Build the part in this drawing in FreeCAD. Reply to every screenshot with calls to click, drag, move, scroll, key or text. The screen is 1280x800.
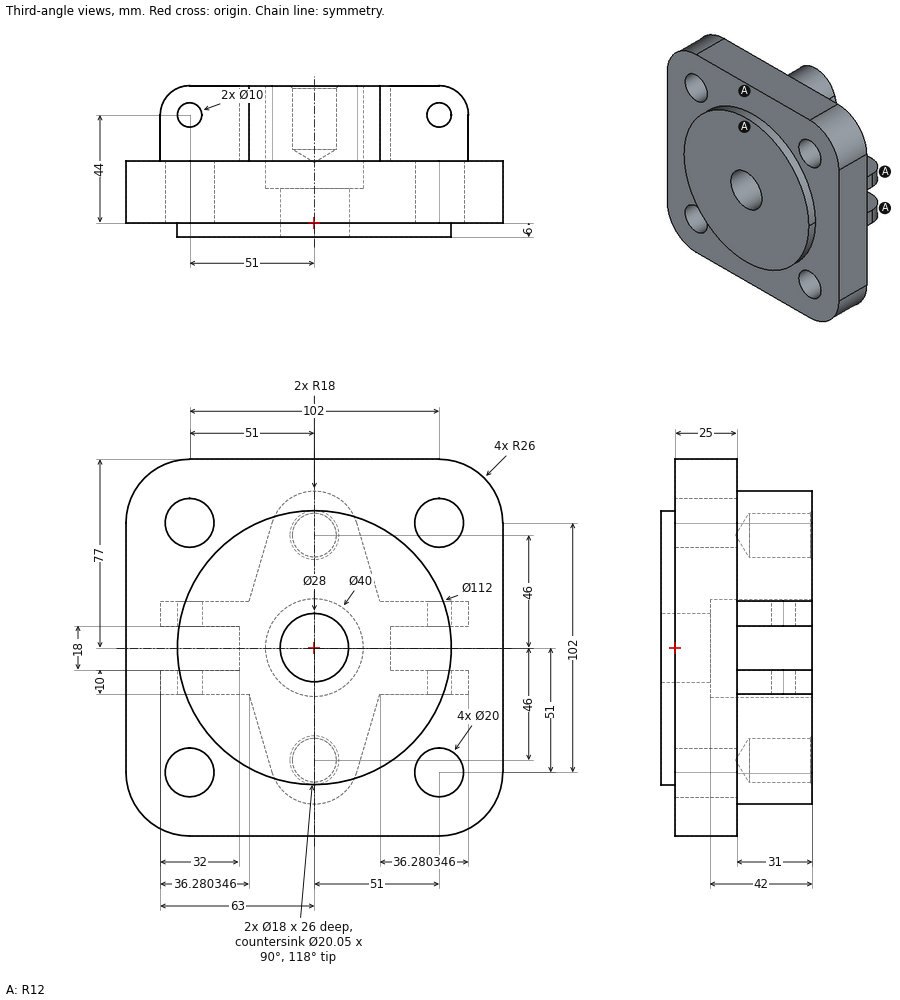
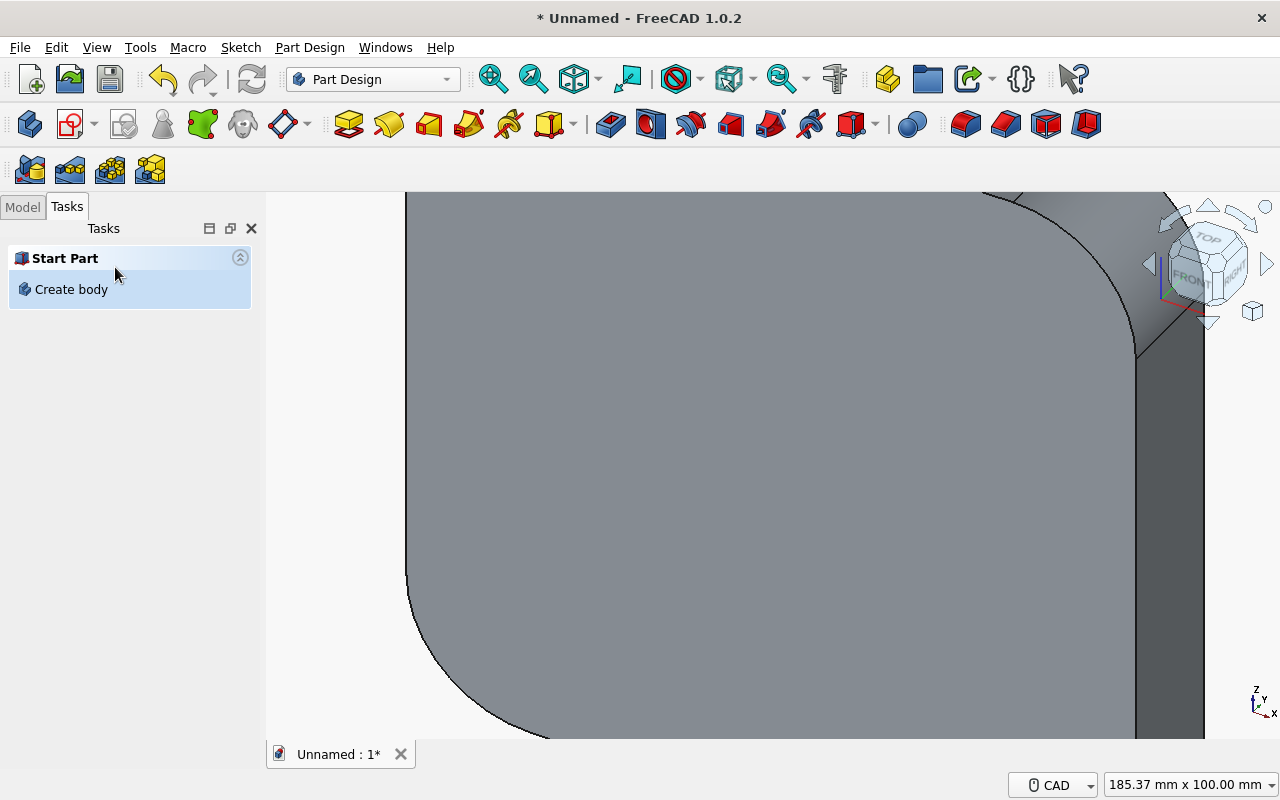
key(v)
key(f)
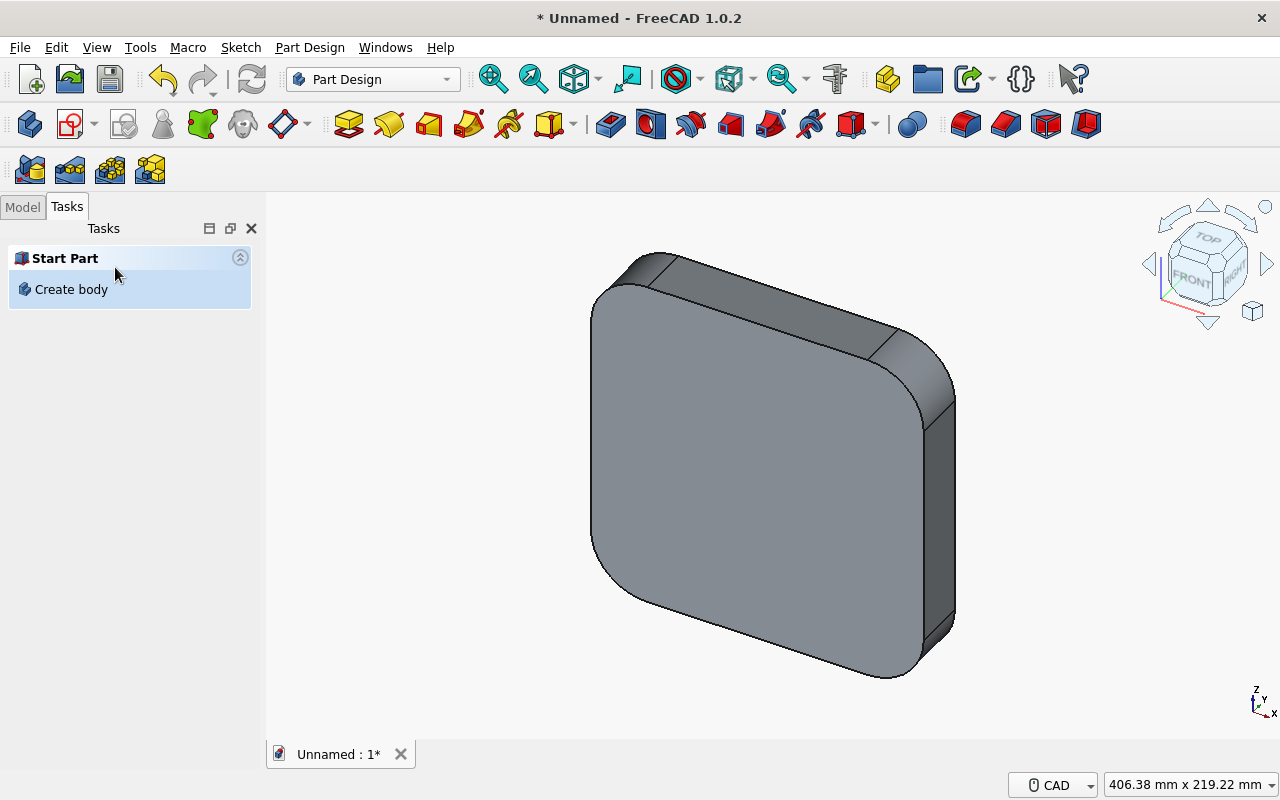
click(70, 124)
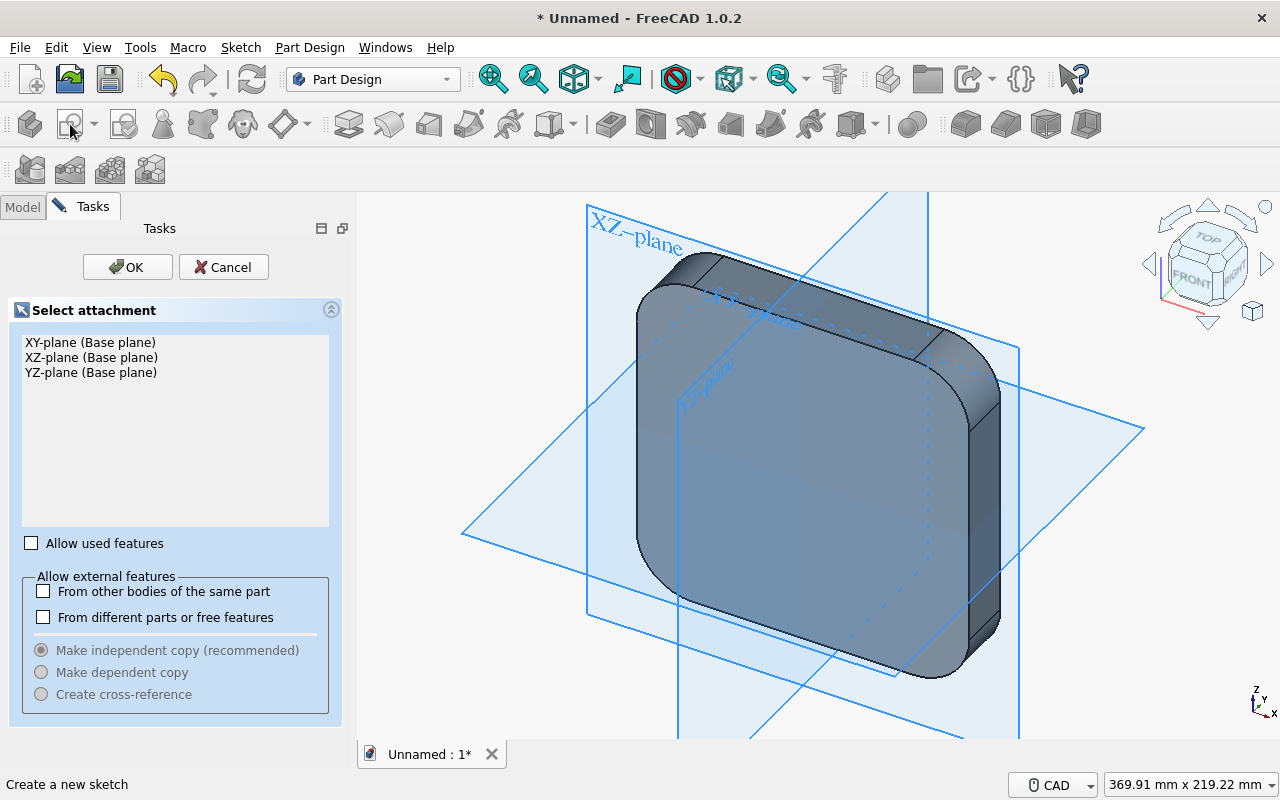
click(82, 358)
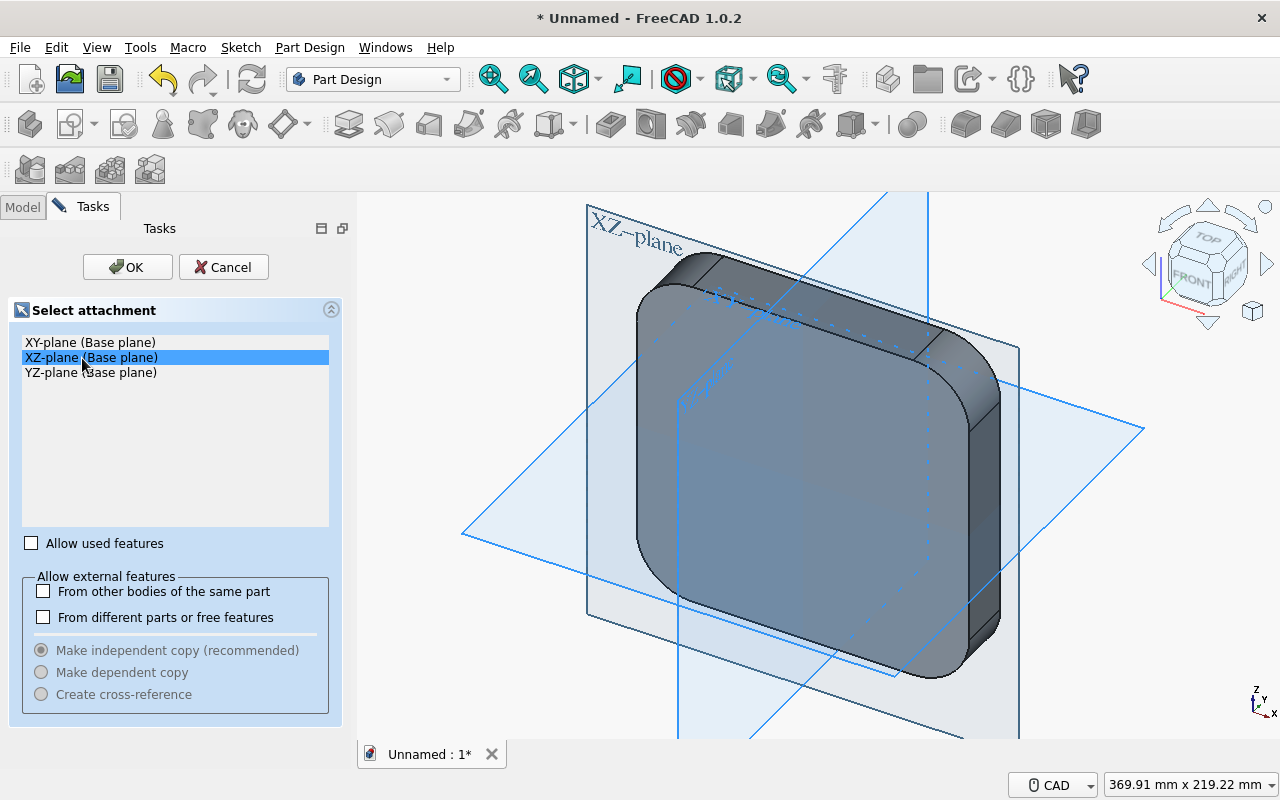
click(128, 267)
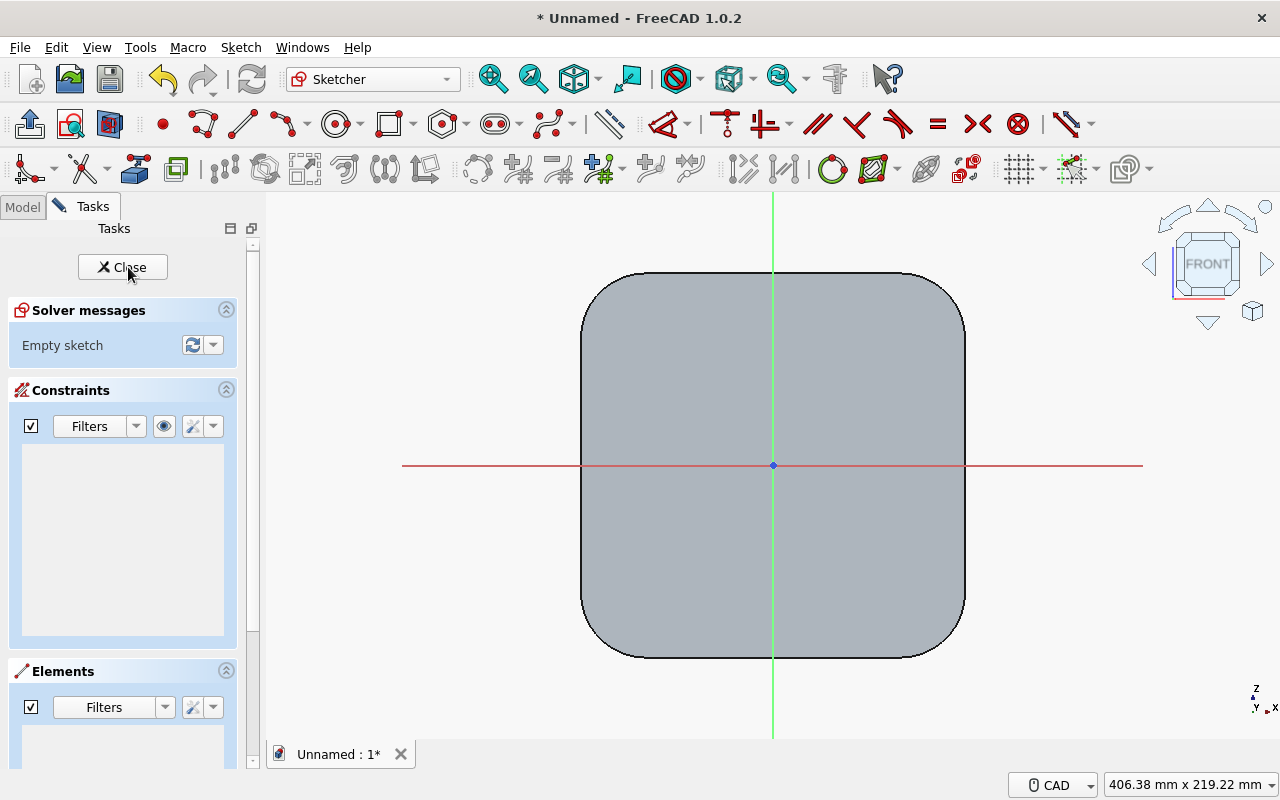
click(336, 124)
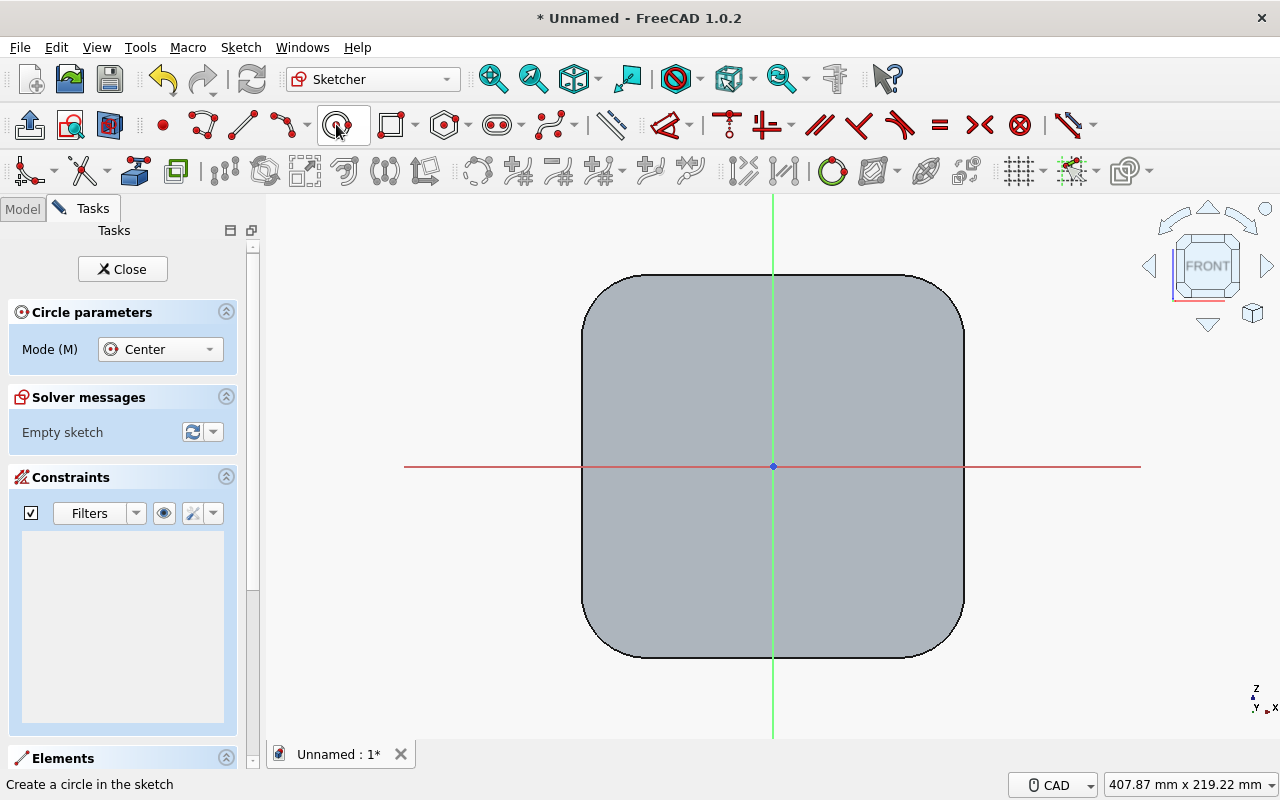
click(773, 466)
click(871, 368)
key(Escape)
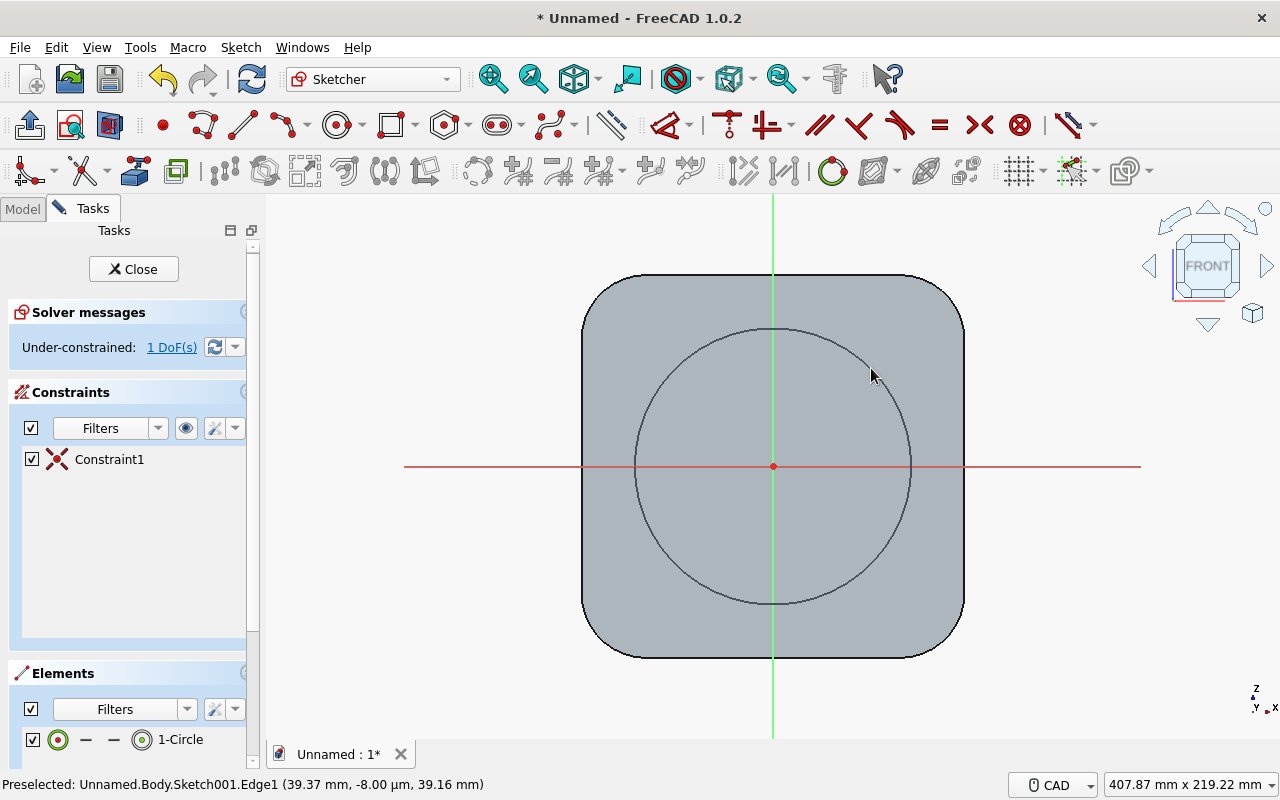
key(d)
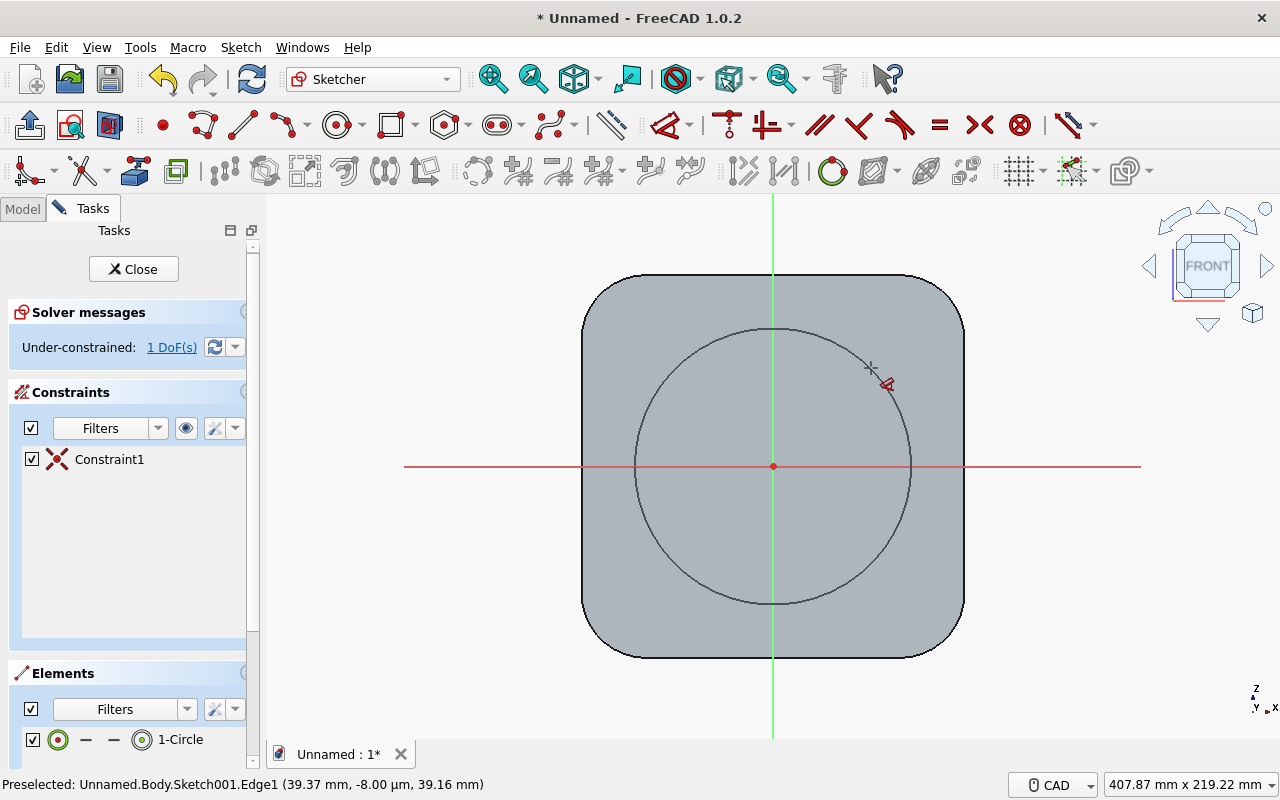
click(870, 368)
click(892, 345)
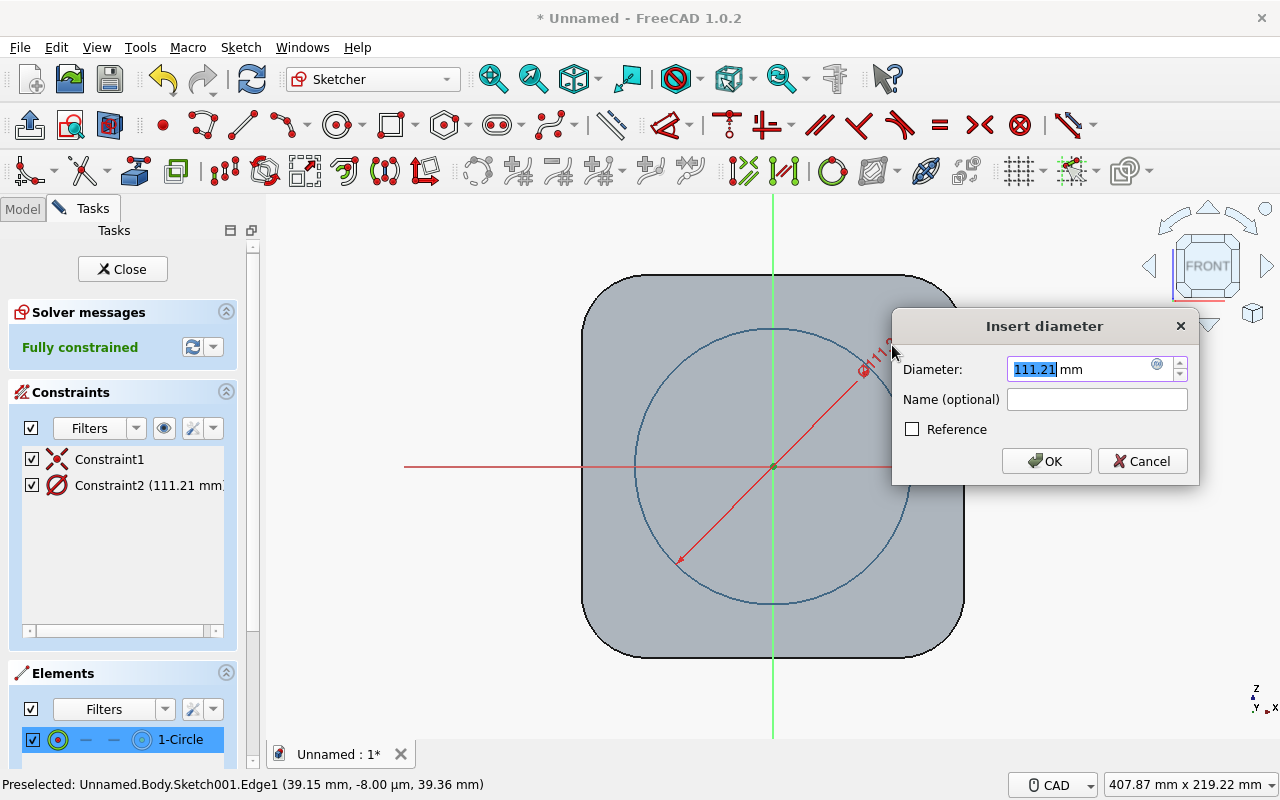
text(112)
key(Return)
key(Escape)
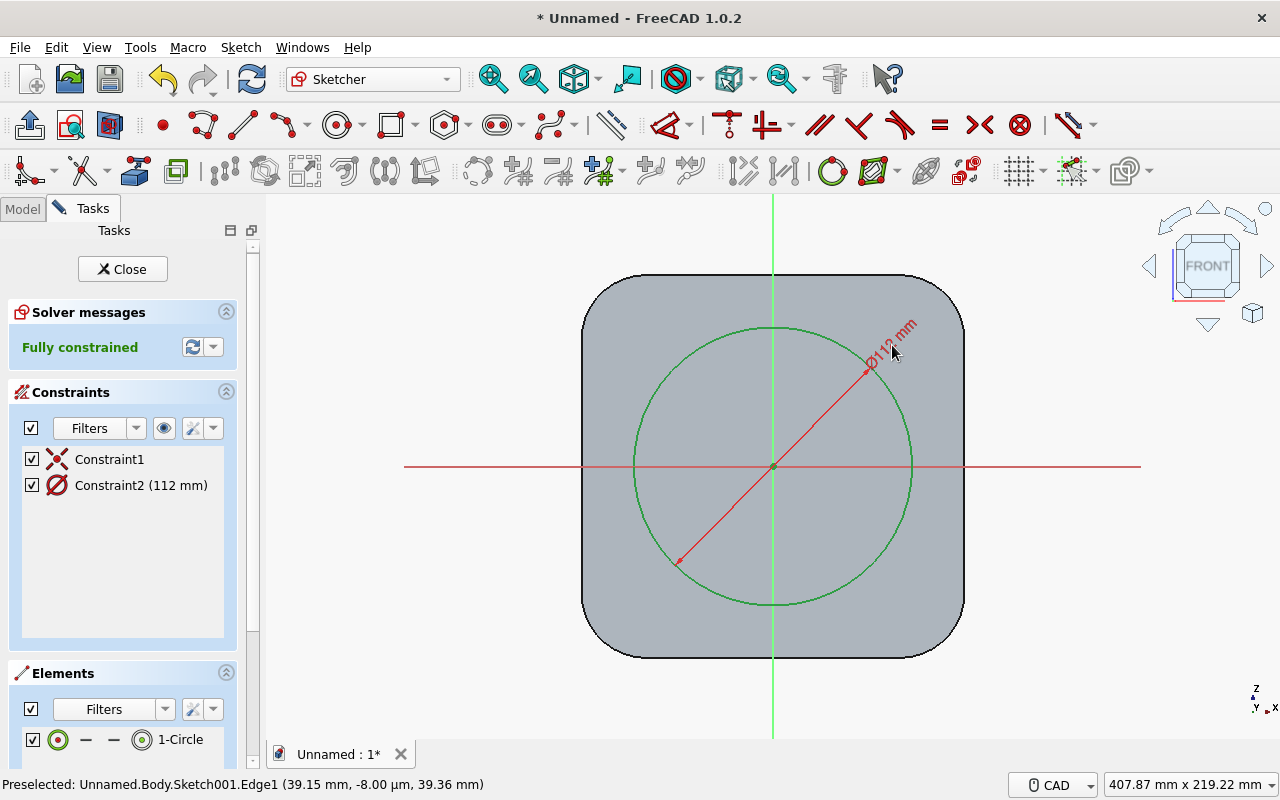
click(123, 269)